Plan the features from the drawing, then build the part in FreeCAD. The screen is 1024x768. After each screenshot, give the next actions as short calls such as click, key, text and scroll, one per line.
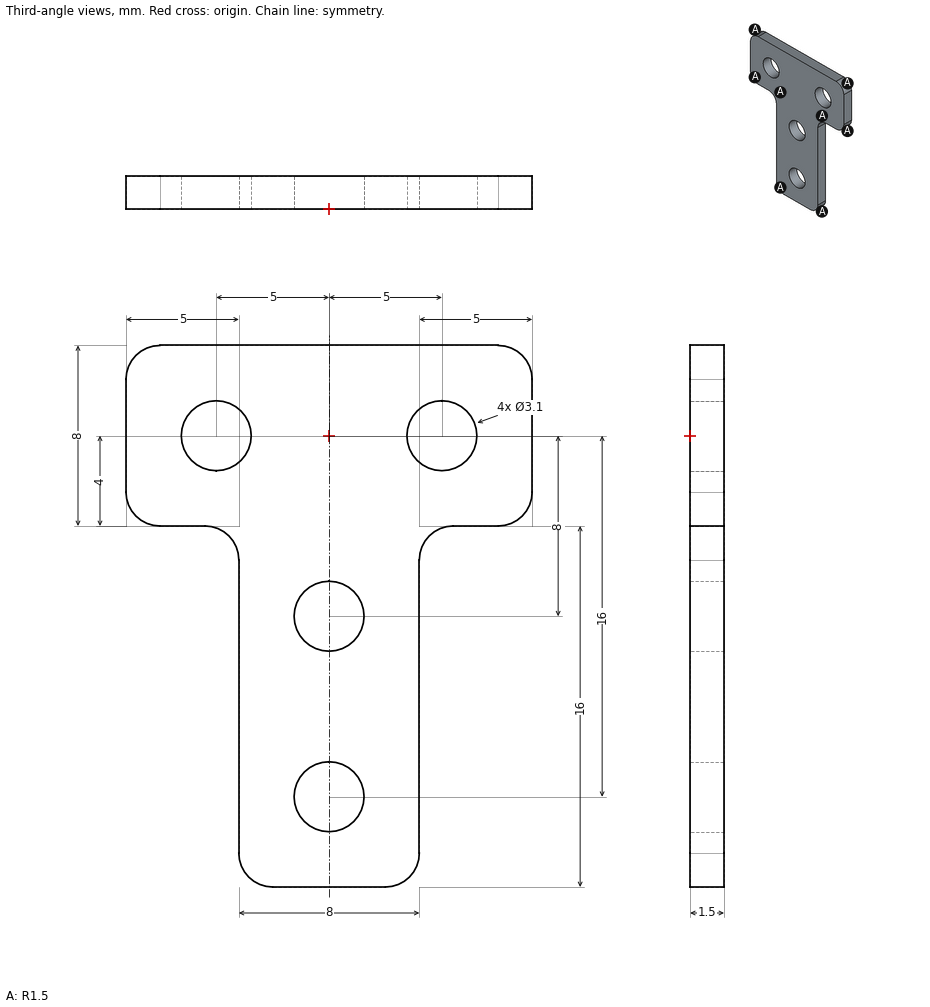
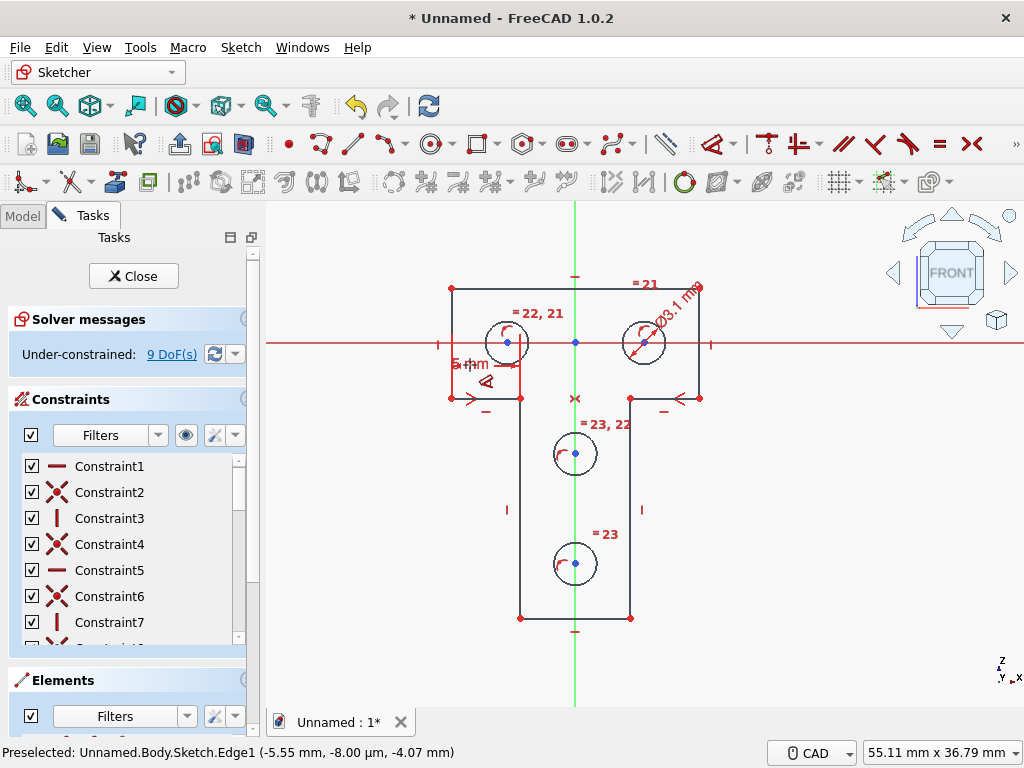
click(452, 366)
click(418, 319)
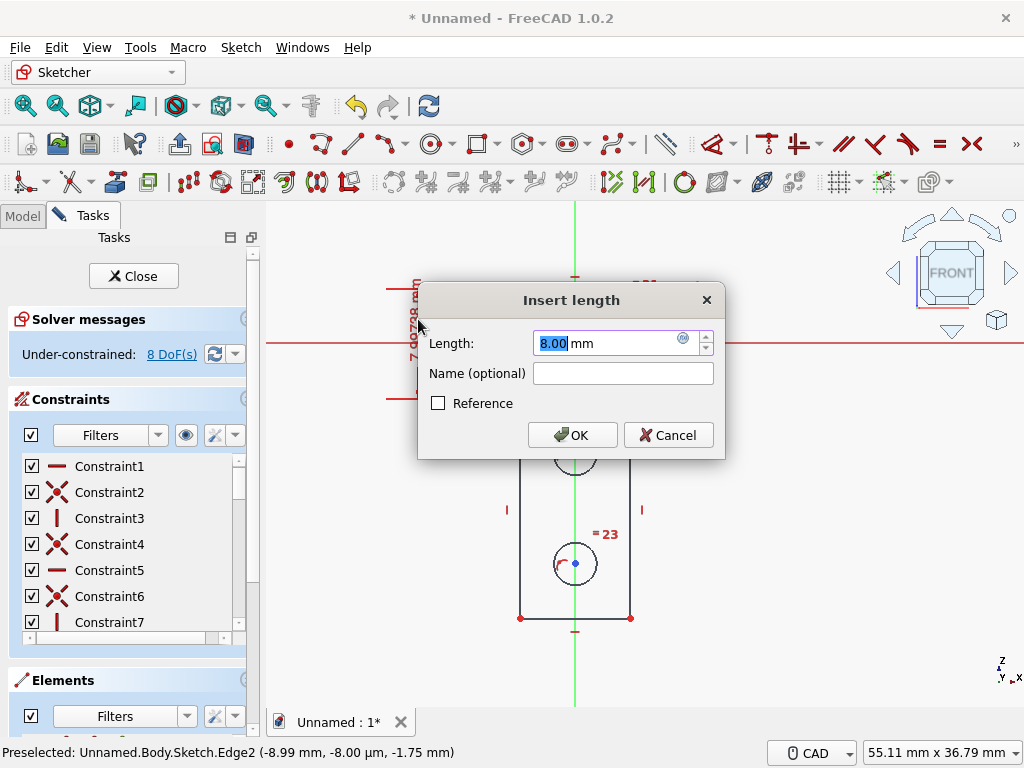
text(8)
key(Return)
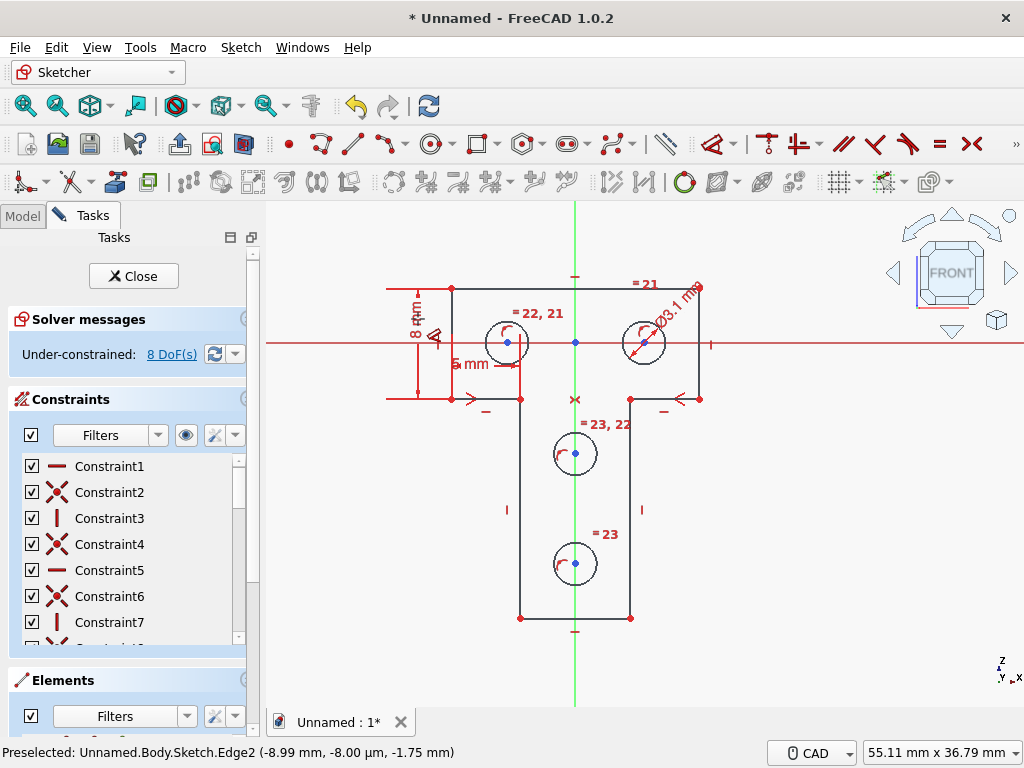
click(678, 399)
click(680, 365)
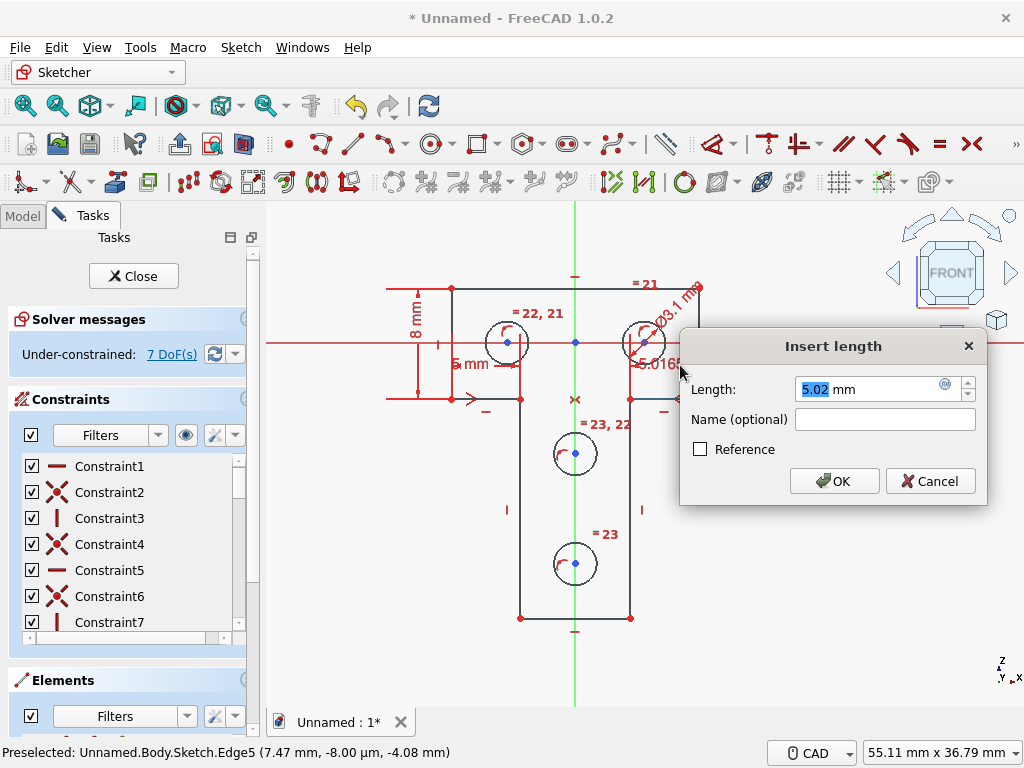
text(5)
key(Return)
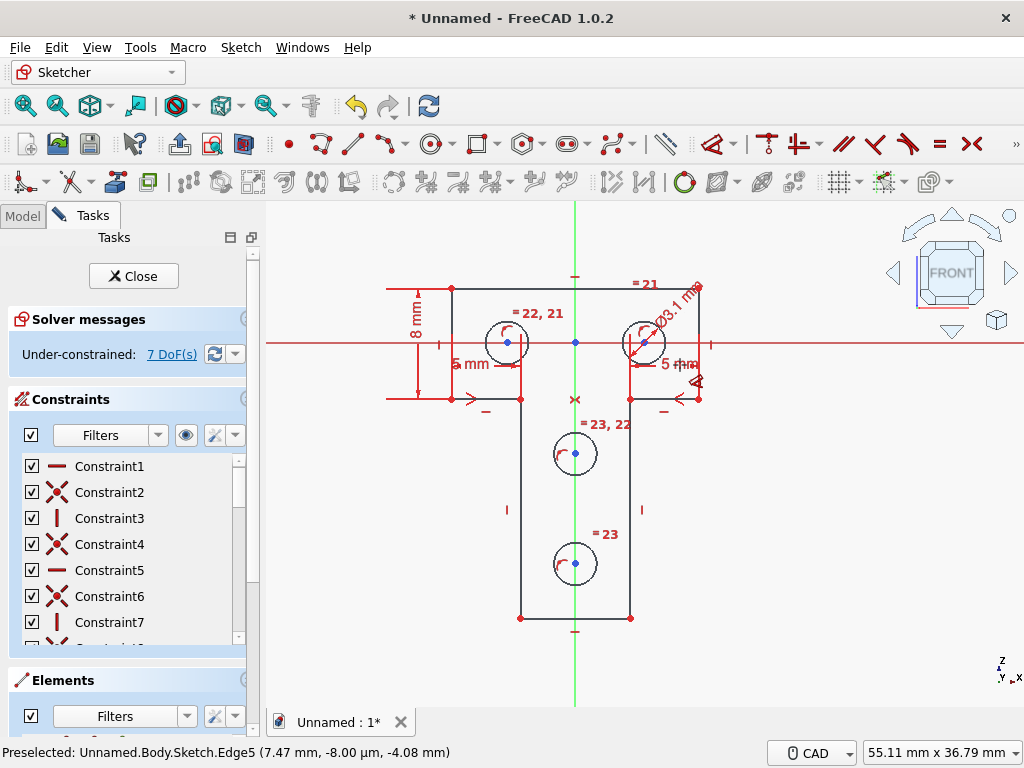
click(597, 619)
click(550, 653)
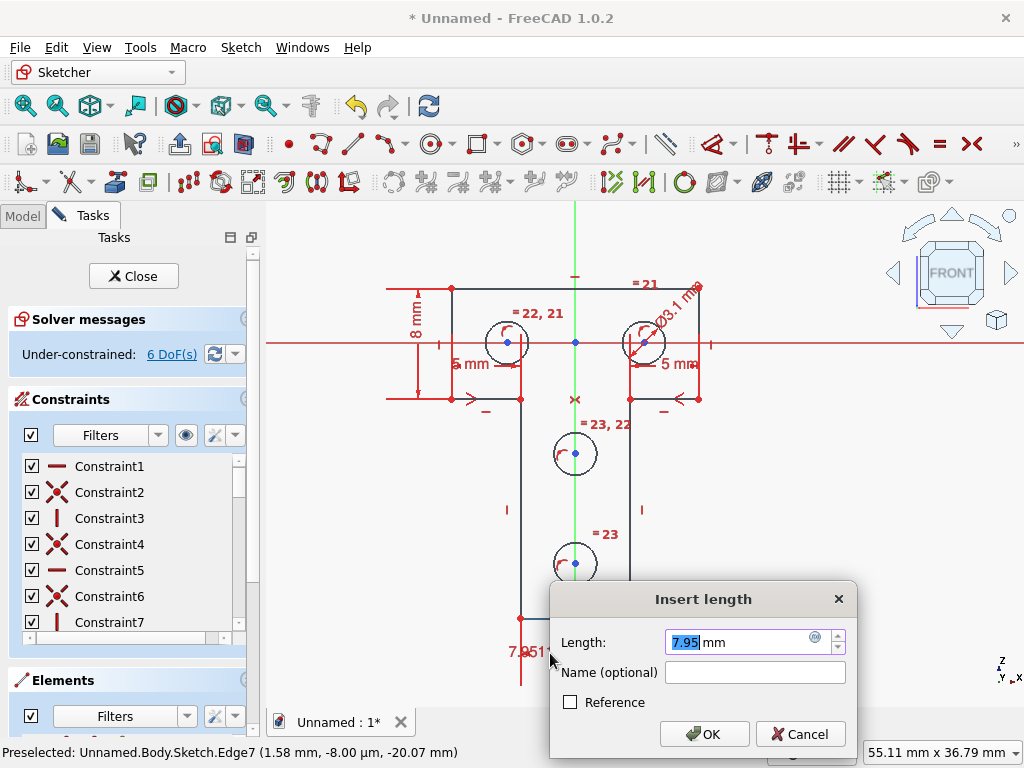
text(8)
key(Return)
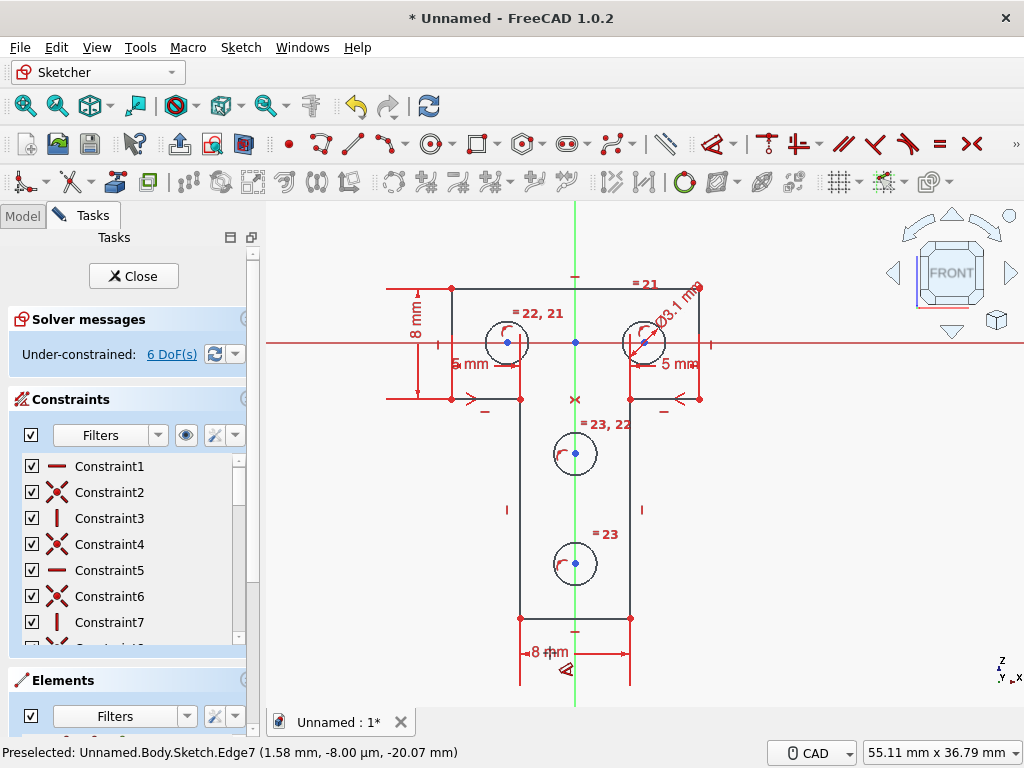
click(644, 343)
click(610, 309)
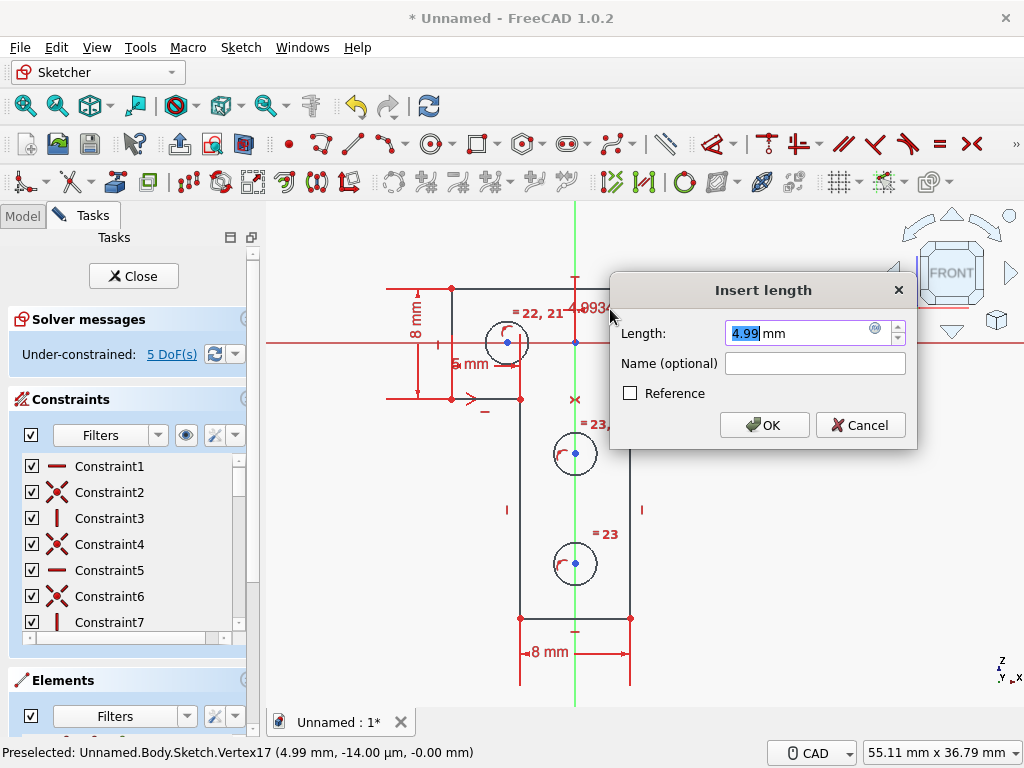
text(5)
key(Return)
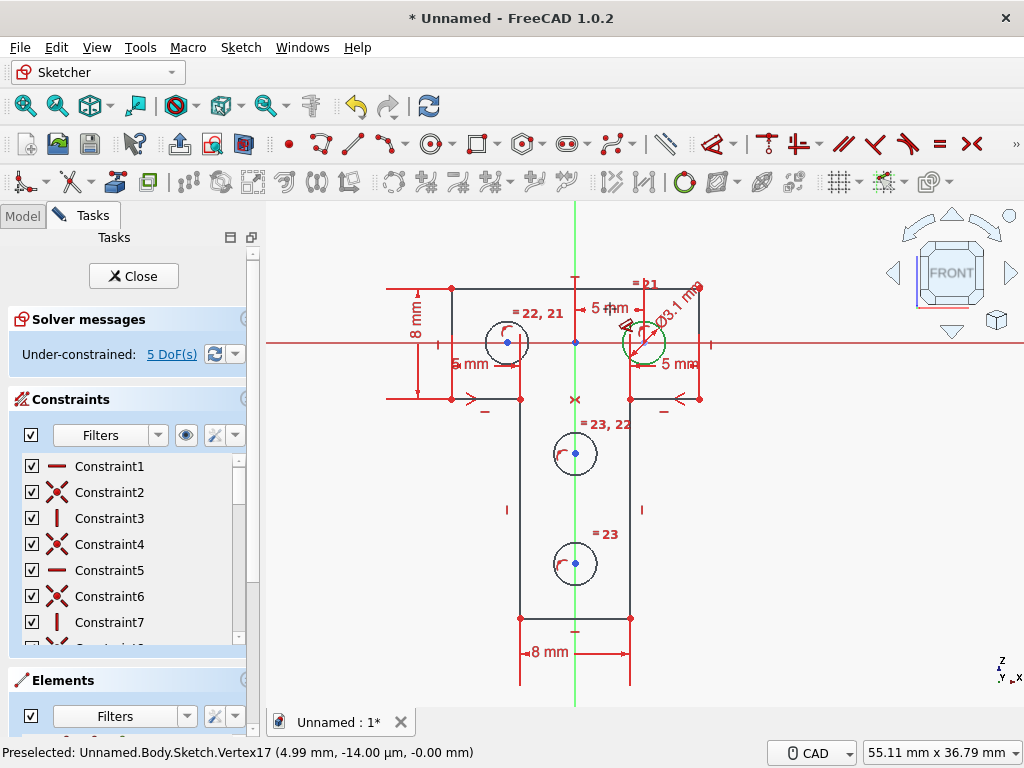
click(507, 343)
click(525, 309)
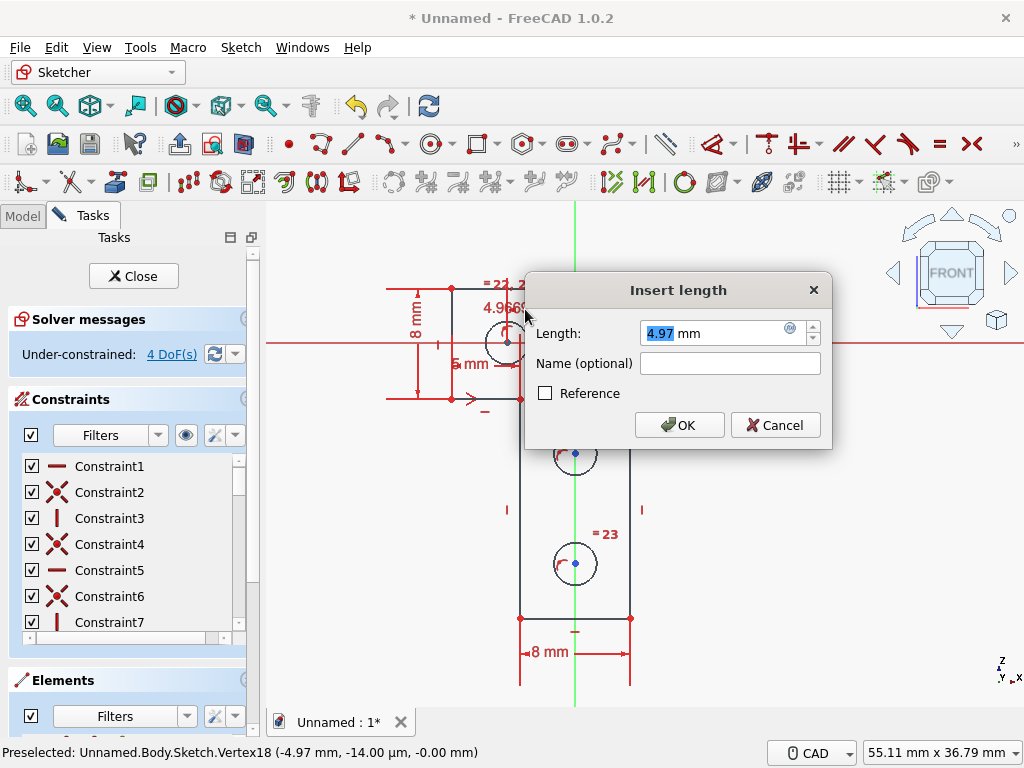
text(5)
key(Return)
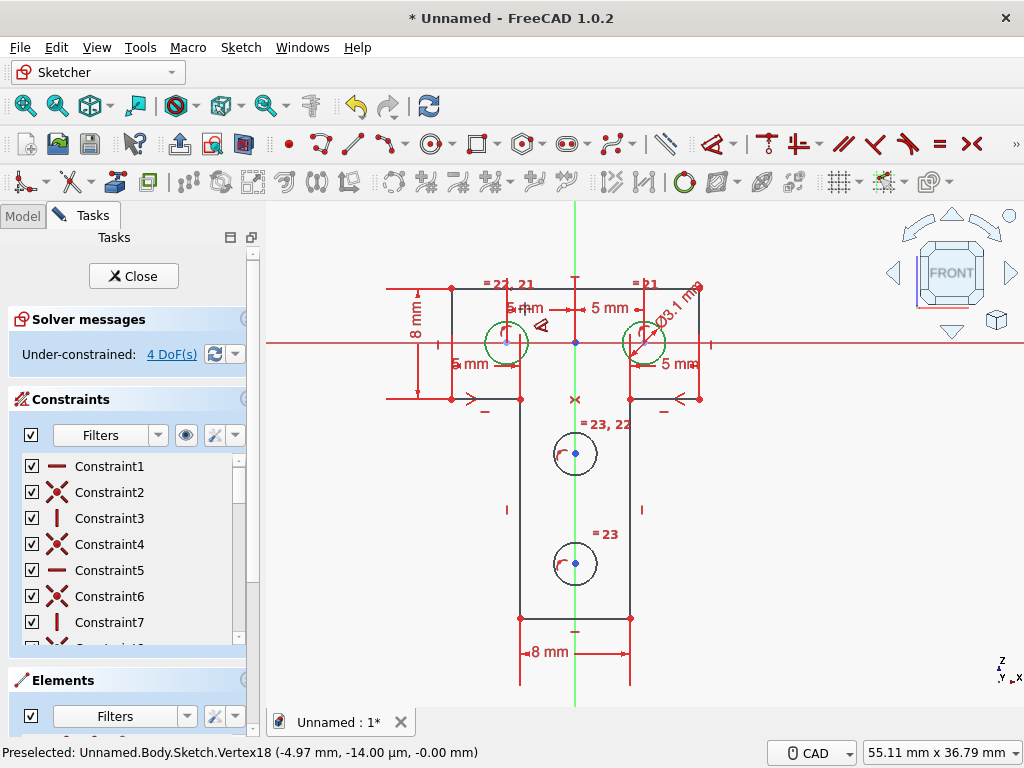
click(575, 454)
click(609, 398)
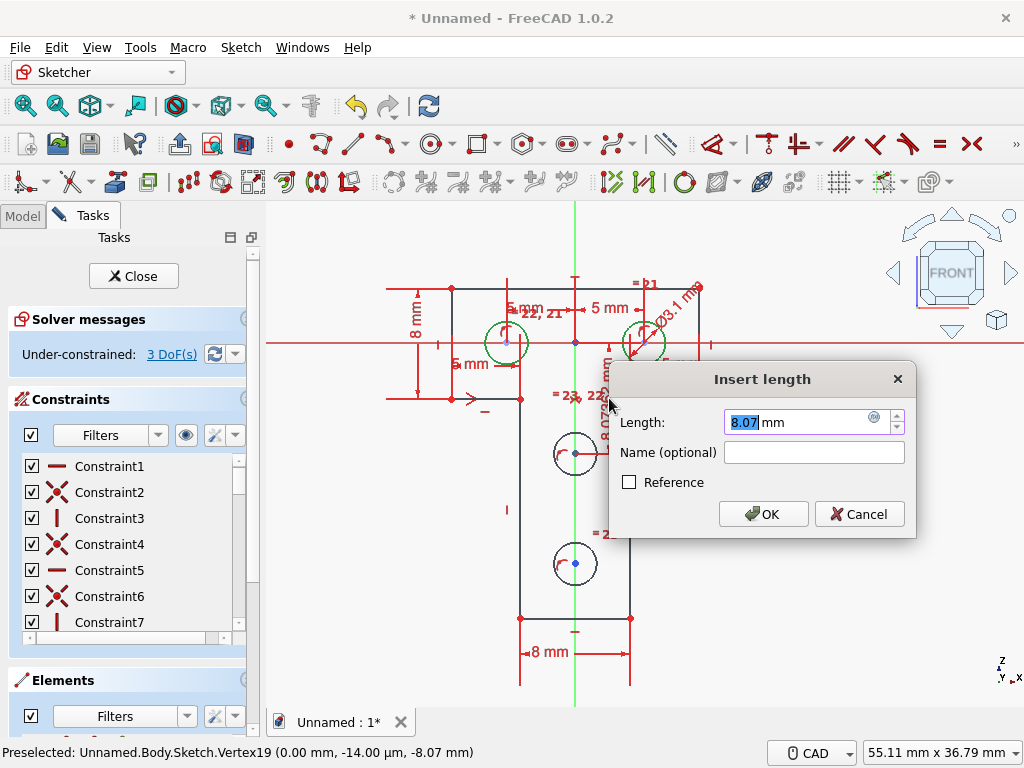
text(8)
key(Return)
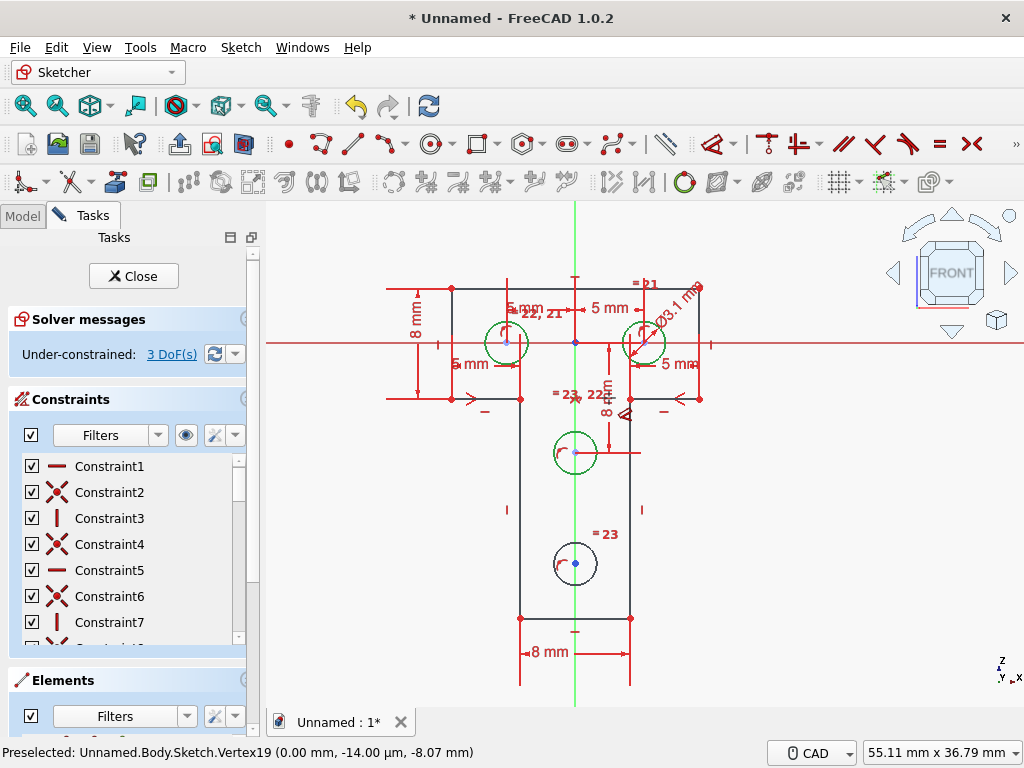
click(630, 465)
click(664, 509)